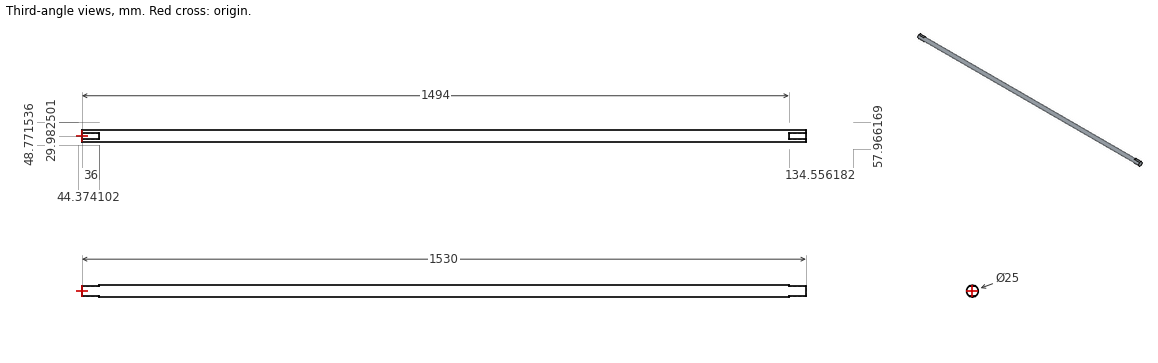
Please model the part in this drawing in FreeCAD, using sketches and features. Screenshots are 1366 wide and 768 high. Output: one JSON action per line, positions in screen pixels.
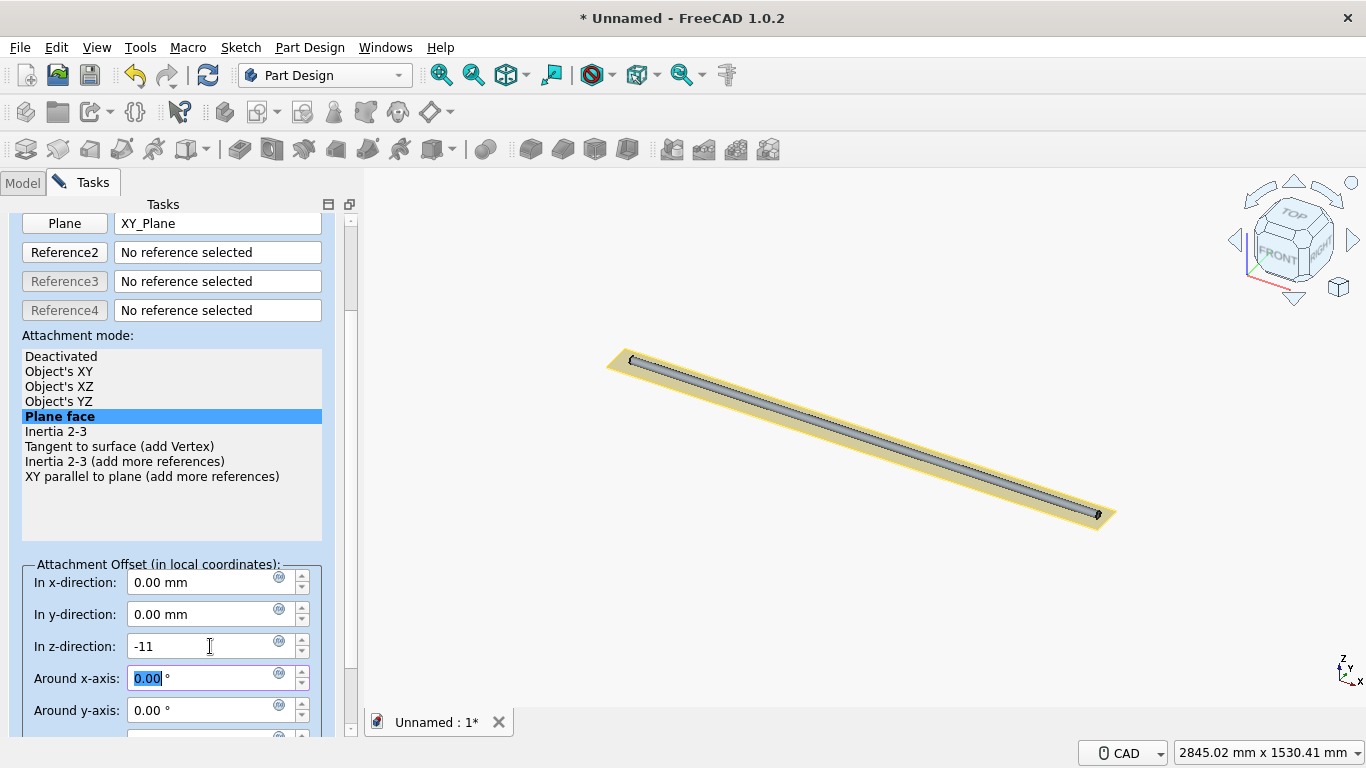
{"action": "scroll", "coordinate": [351, 475], "scroll_direction": "up", "scroll_amount": 3}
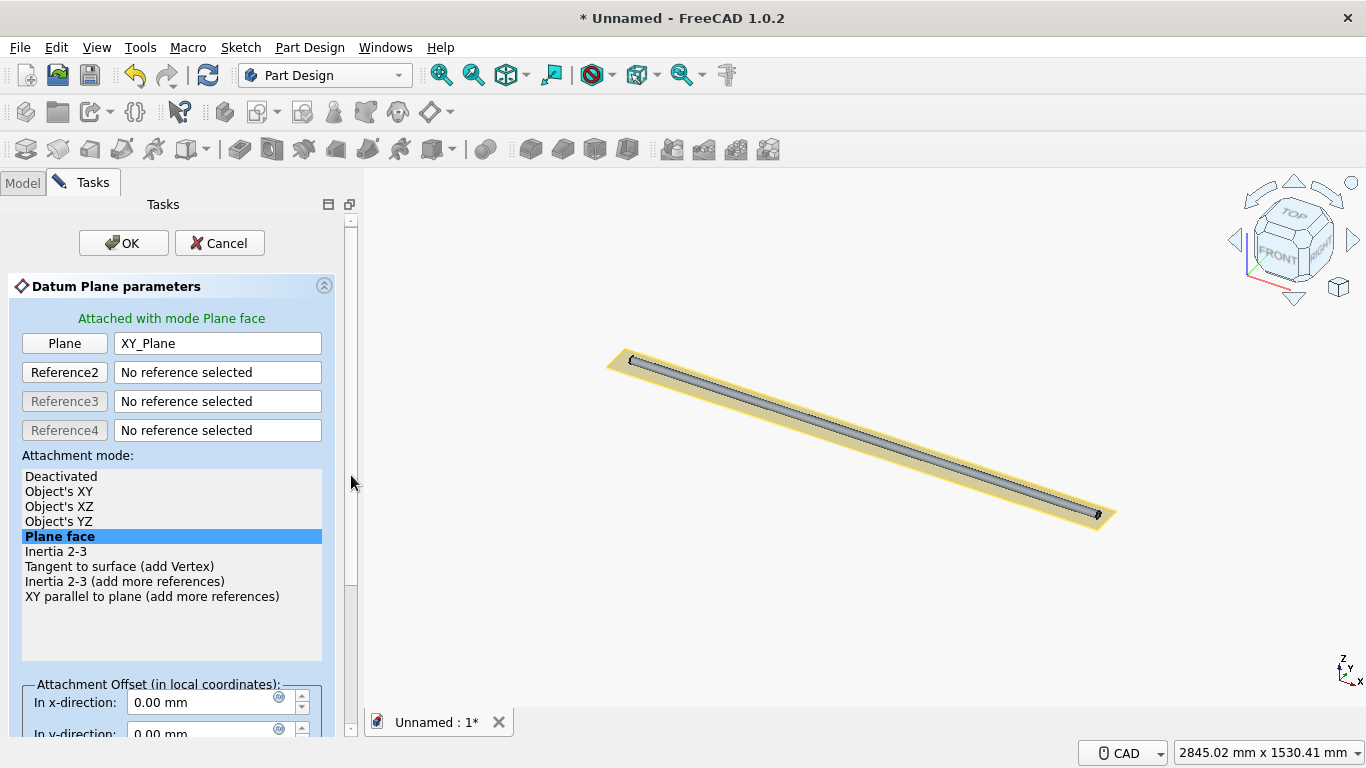
{"action": "left_click", "coordinate": [124, 243]}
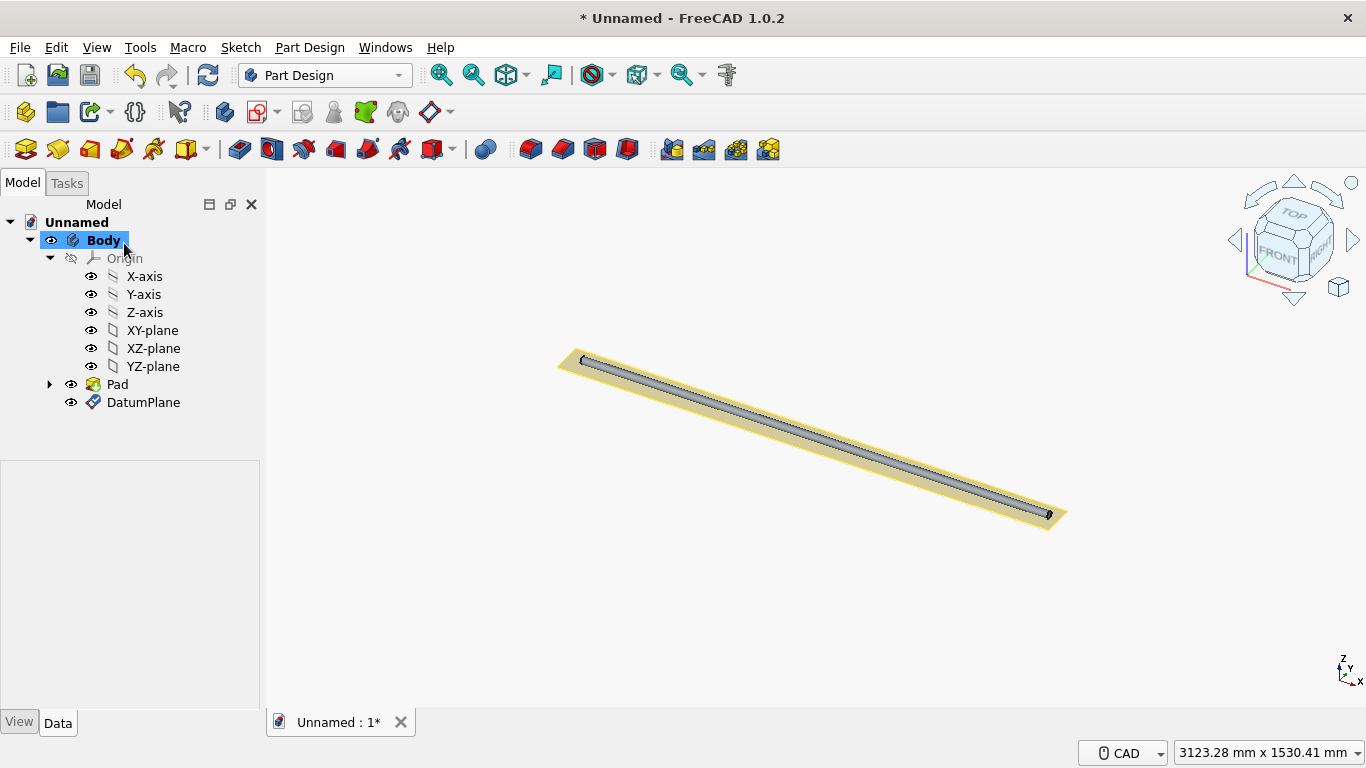
{"action": "left_click", "coordinate": [116, 402]}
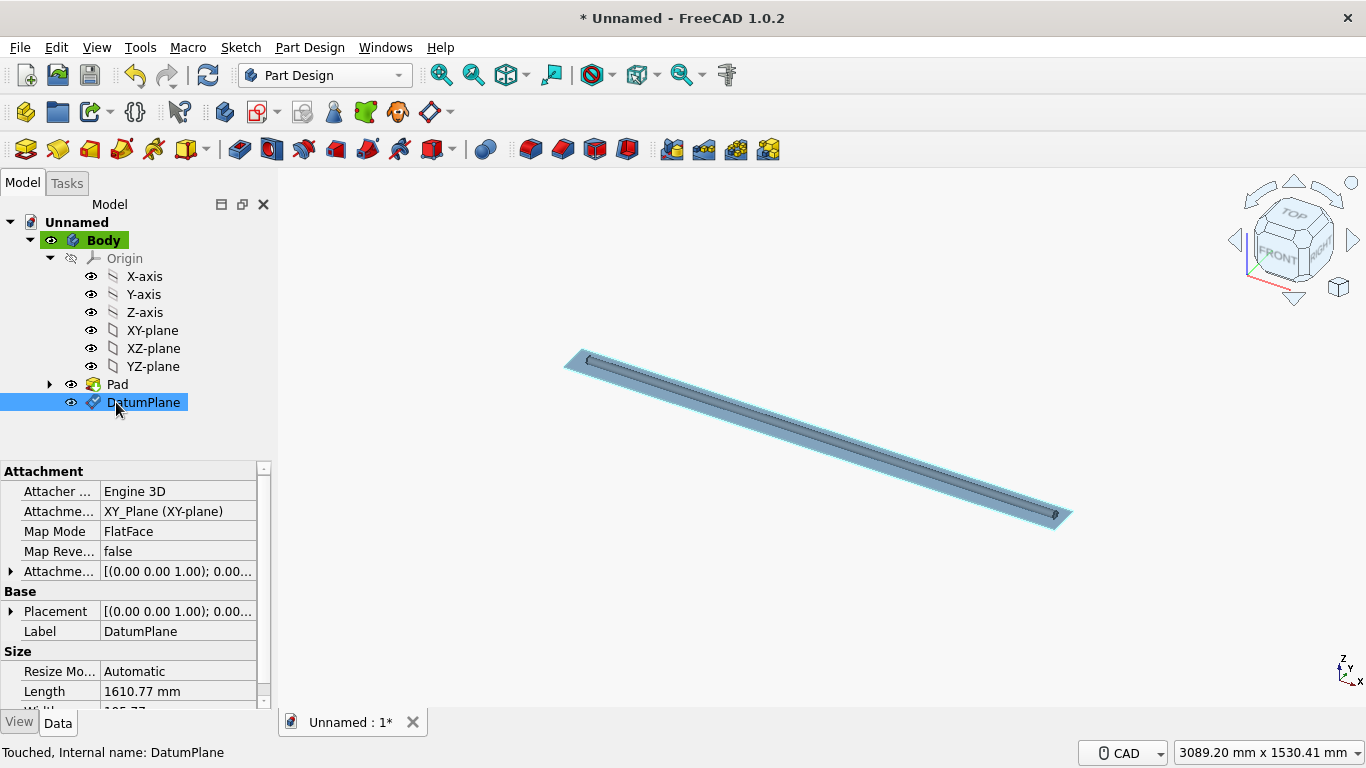
{"action": "left_click", "coordinate": [258, 112]}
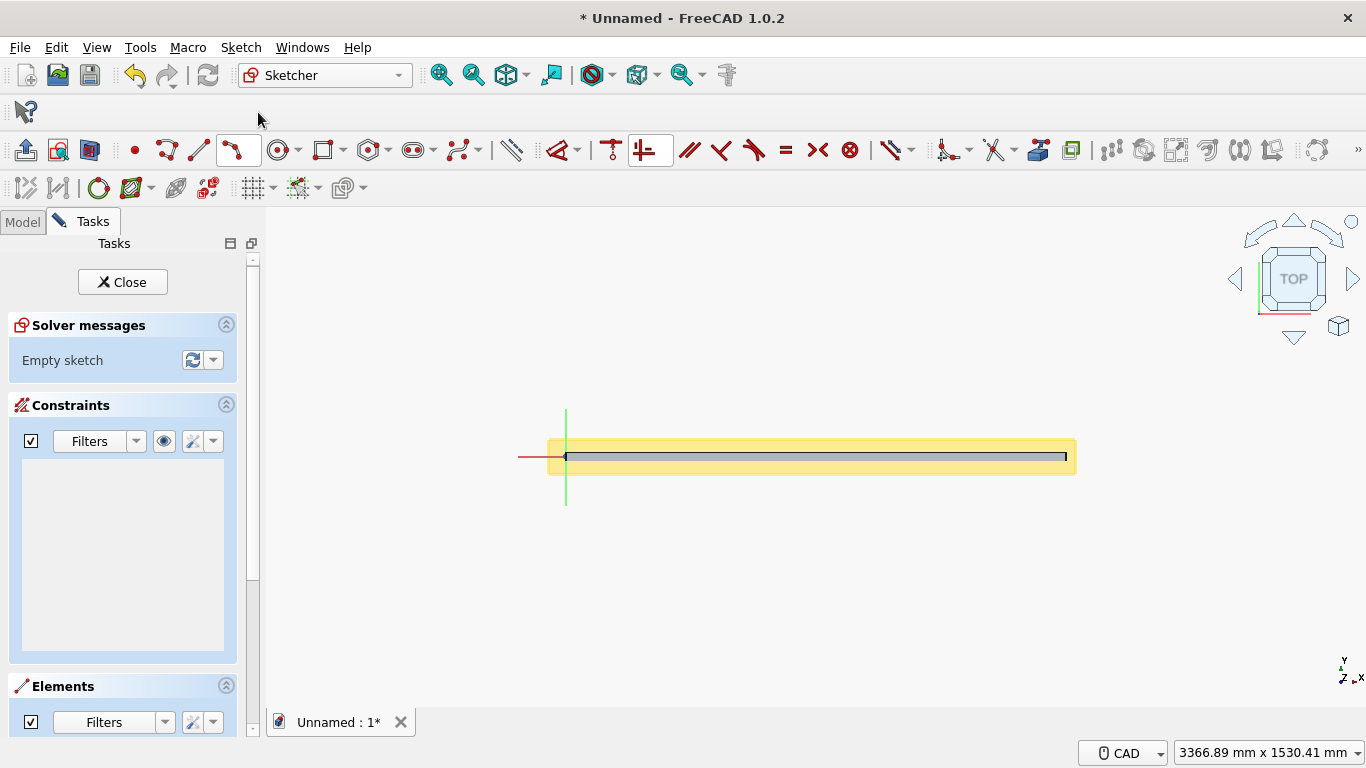
{"action": "left_click", "coordinate": [90, 150]}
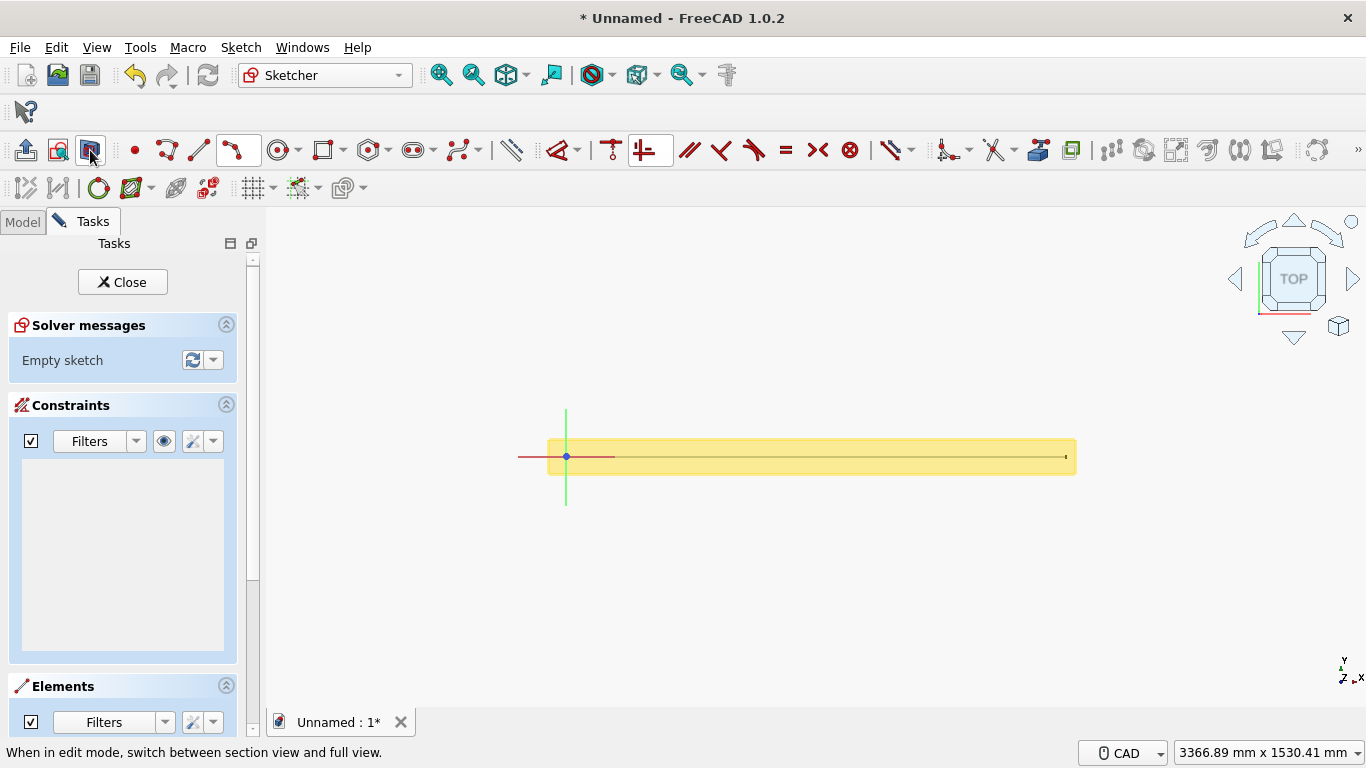
{"action": "left_click", "coordinate": [324, 150]}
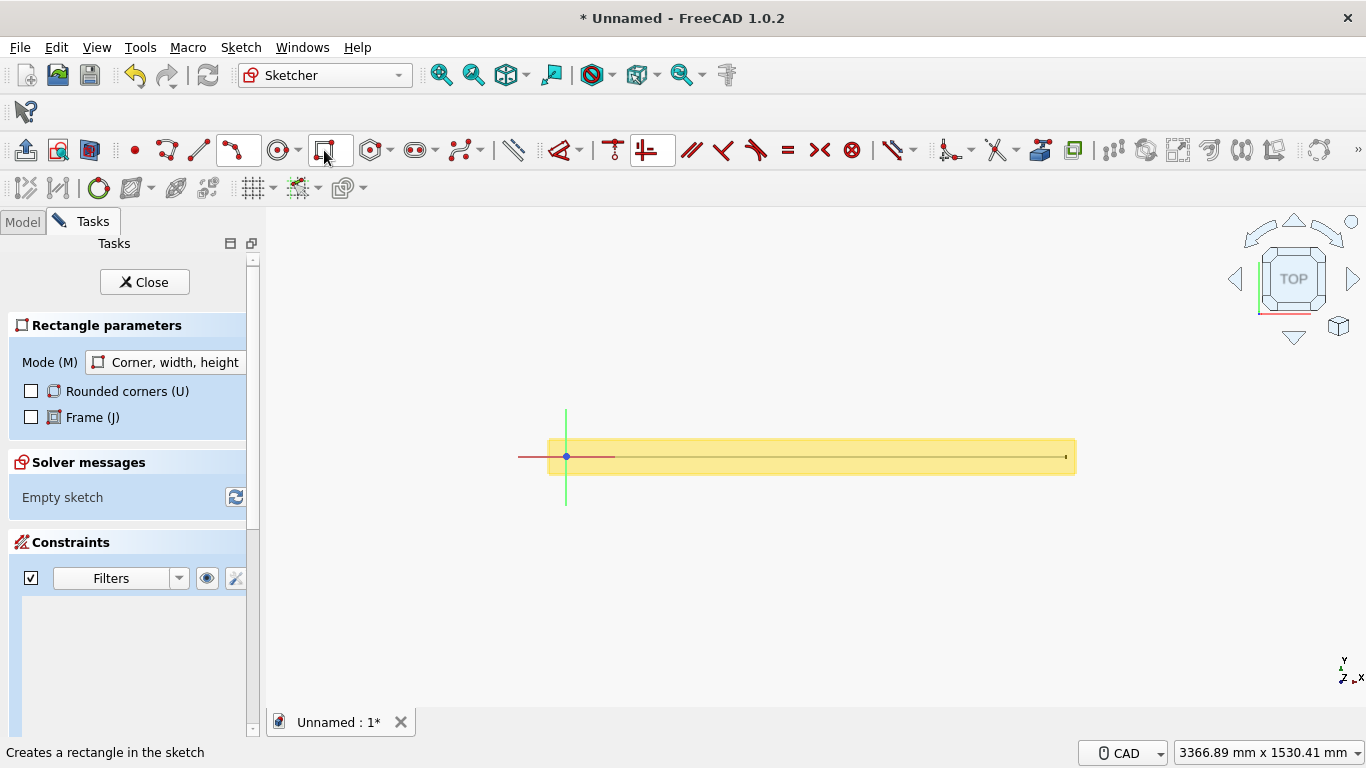
{"action": "scroll", "coordinate": [563, 447], "scroll_direction": "up", "scroll_amount": 9}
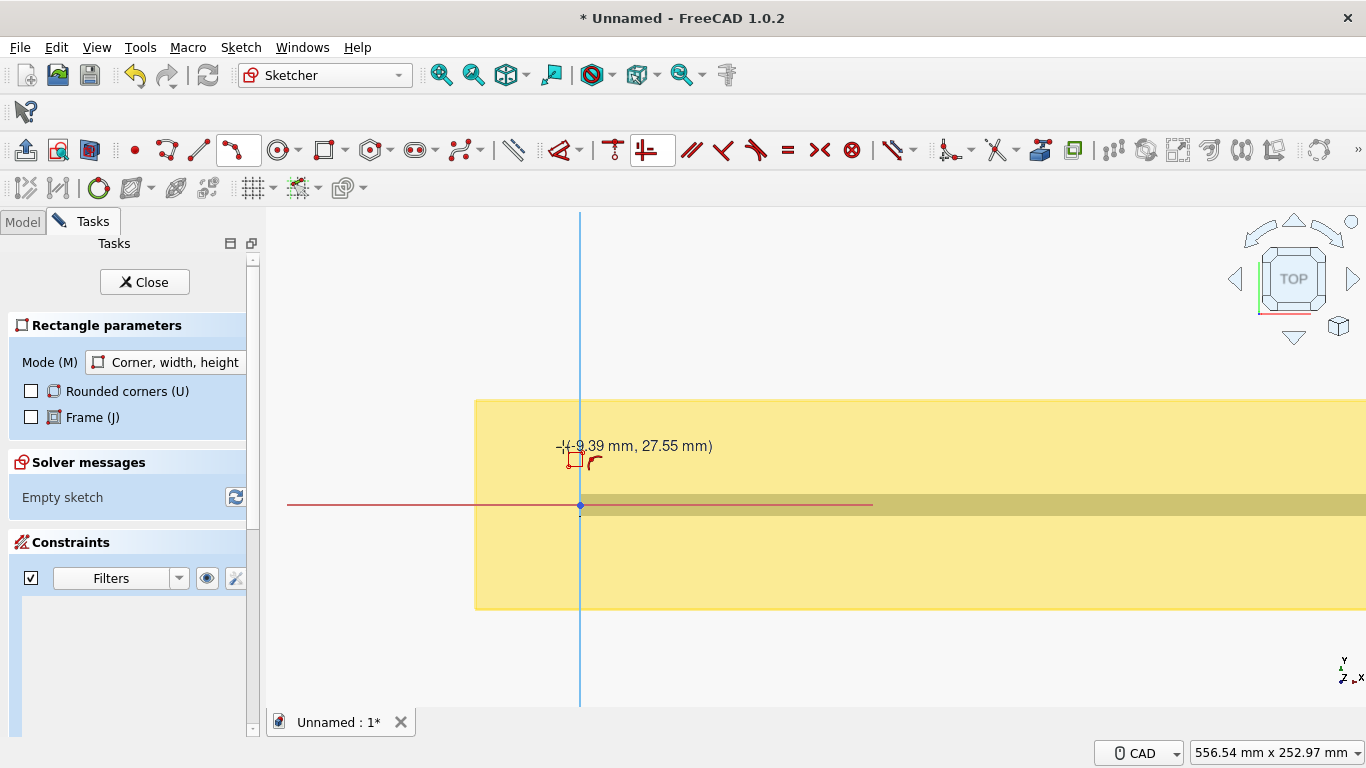
{"action": "left_click", "coordinate": [564, 446]}
{"action": "mouse_move", "coordinate": [651, 542]}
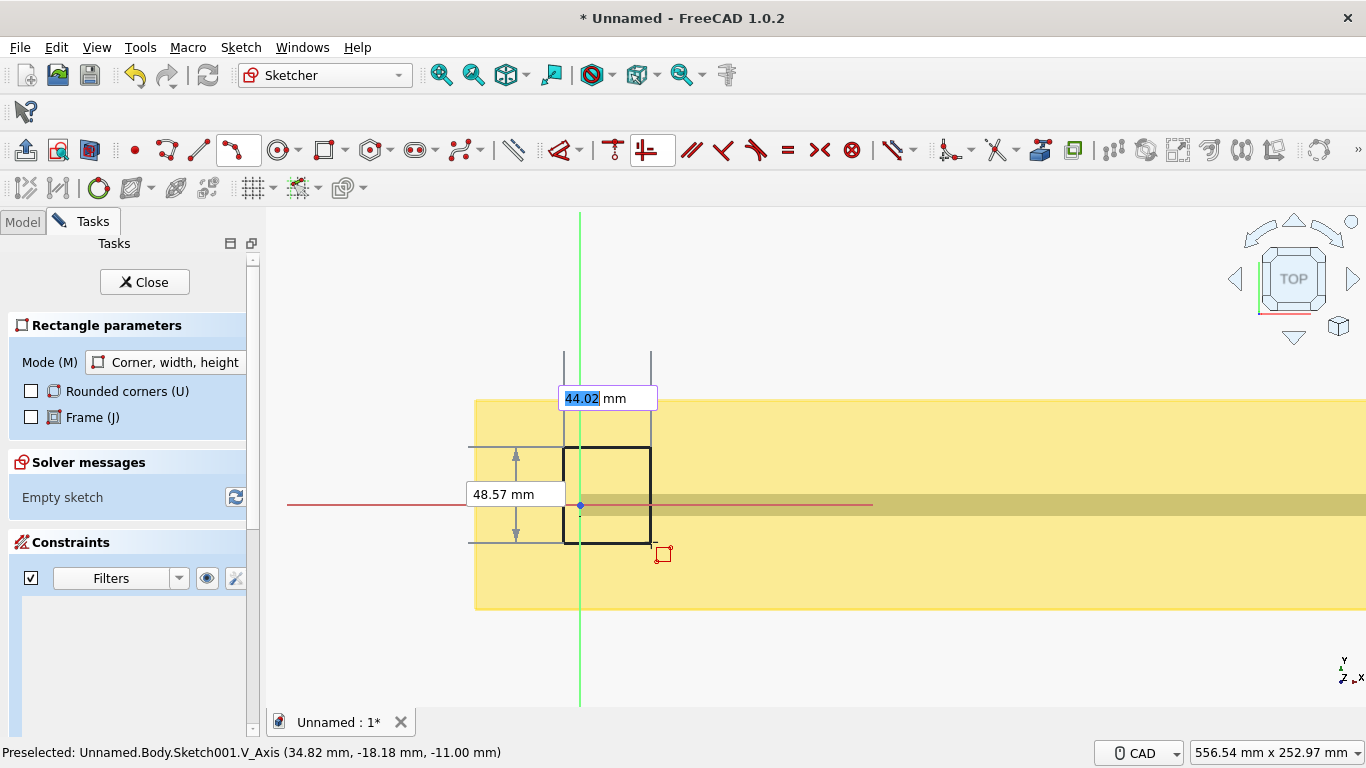
{"action": "type", "text": "44.374102"}
{"action": "key", "text": "Tab"}
{"action": "type", "text": "48.771536"}
{"action": "key", "text": "Return"}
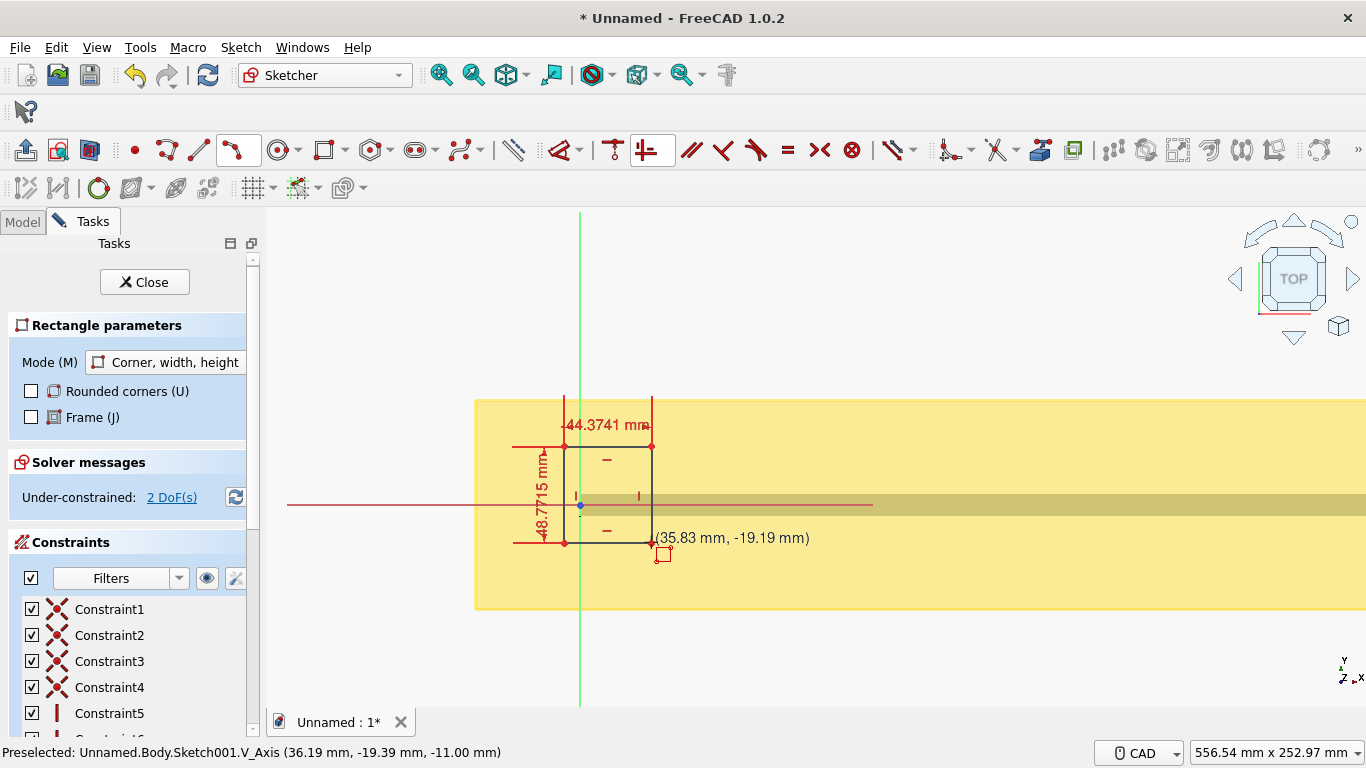
{"action": "scroll", "coordinate": [385, 445], "scroll_direction": "down", "scroll_amount": 8}